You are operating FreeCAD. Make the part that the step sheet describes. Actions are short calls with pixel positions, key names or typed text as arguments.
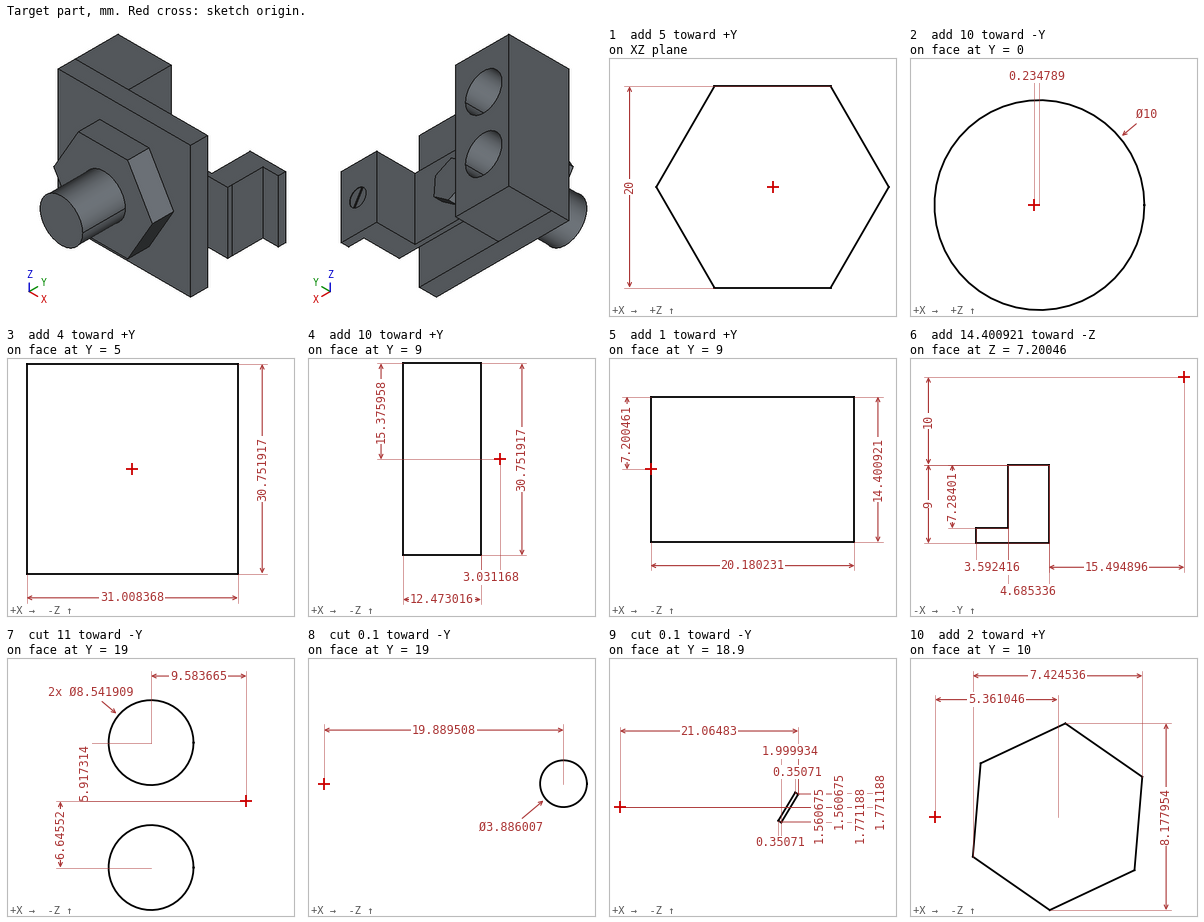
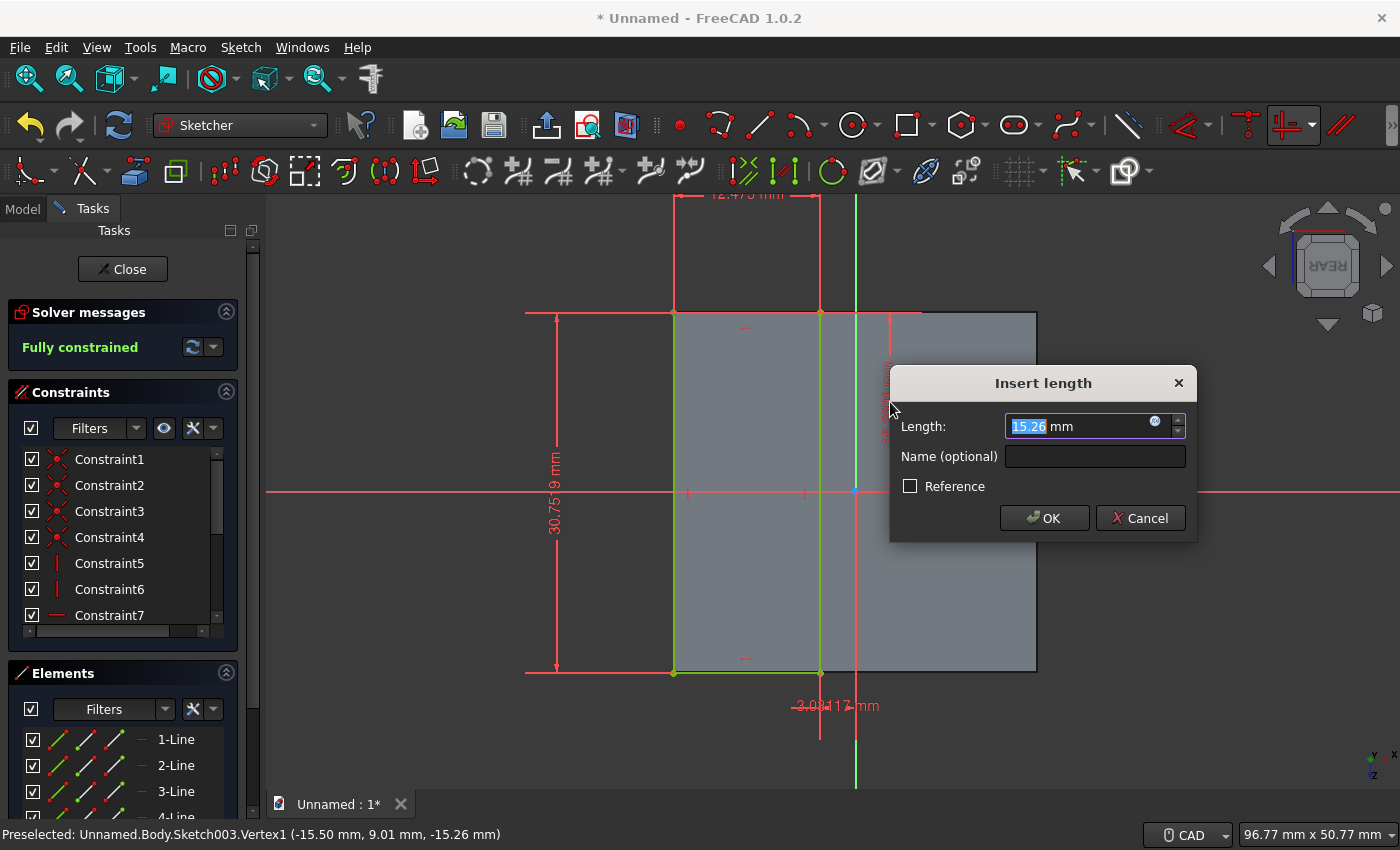
text(15.375958)
key(Return)
key(Escape)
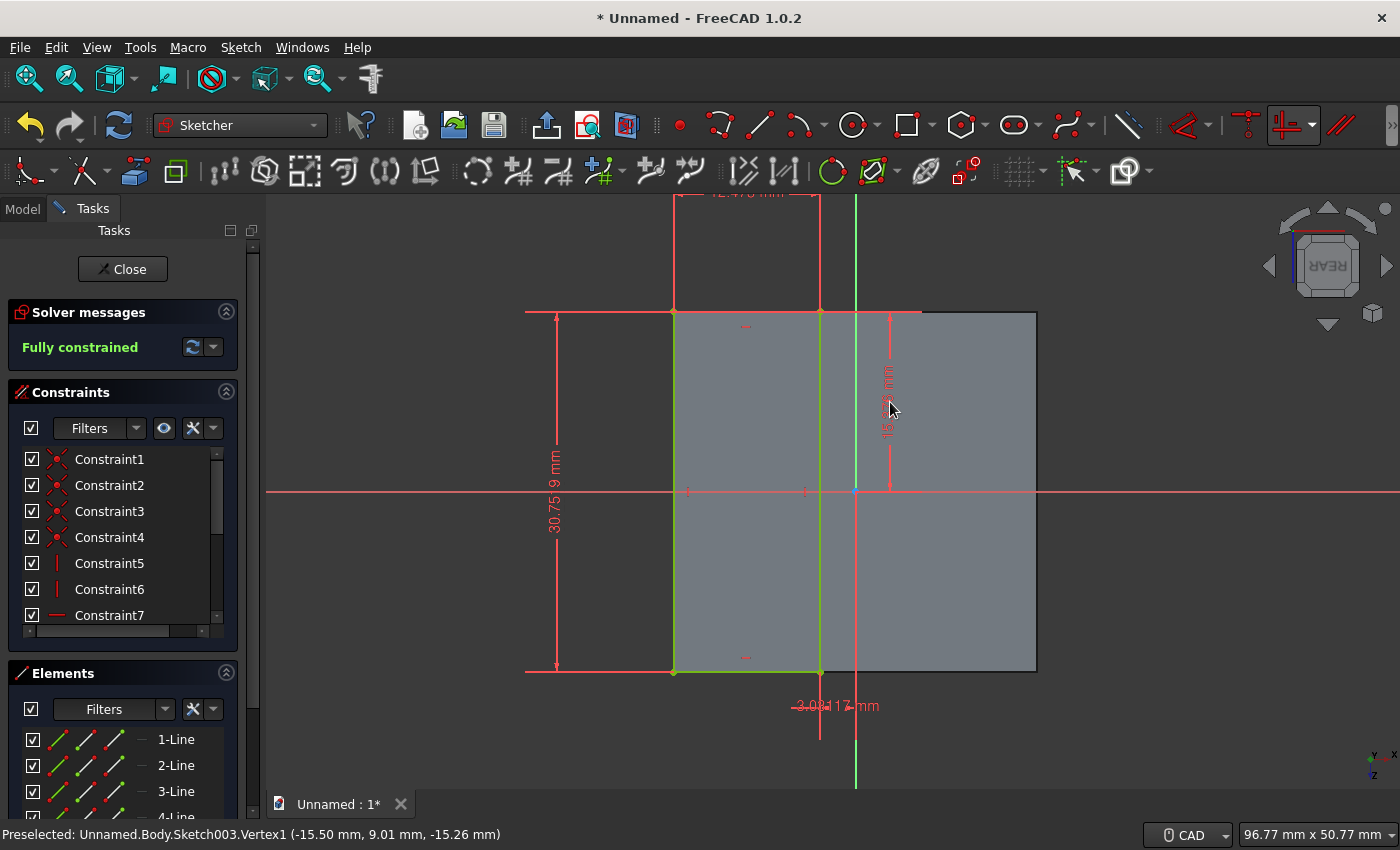
click(123, 269)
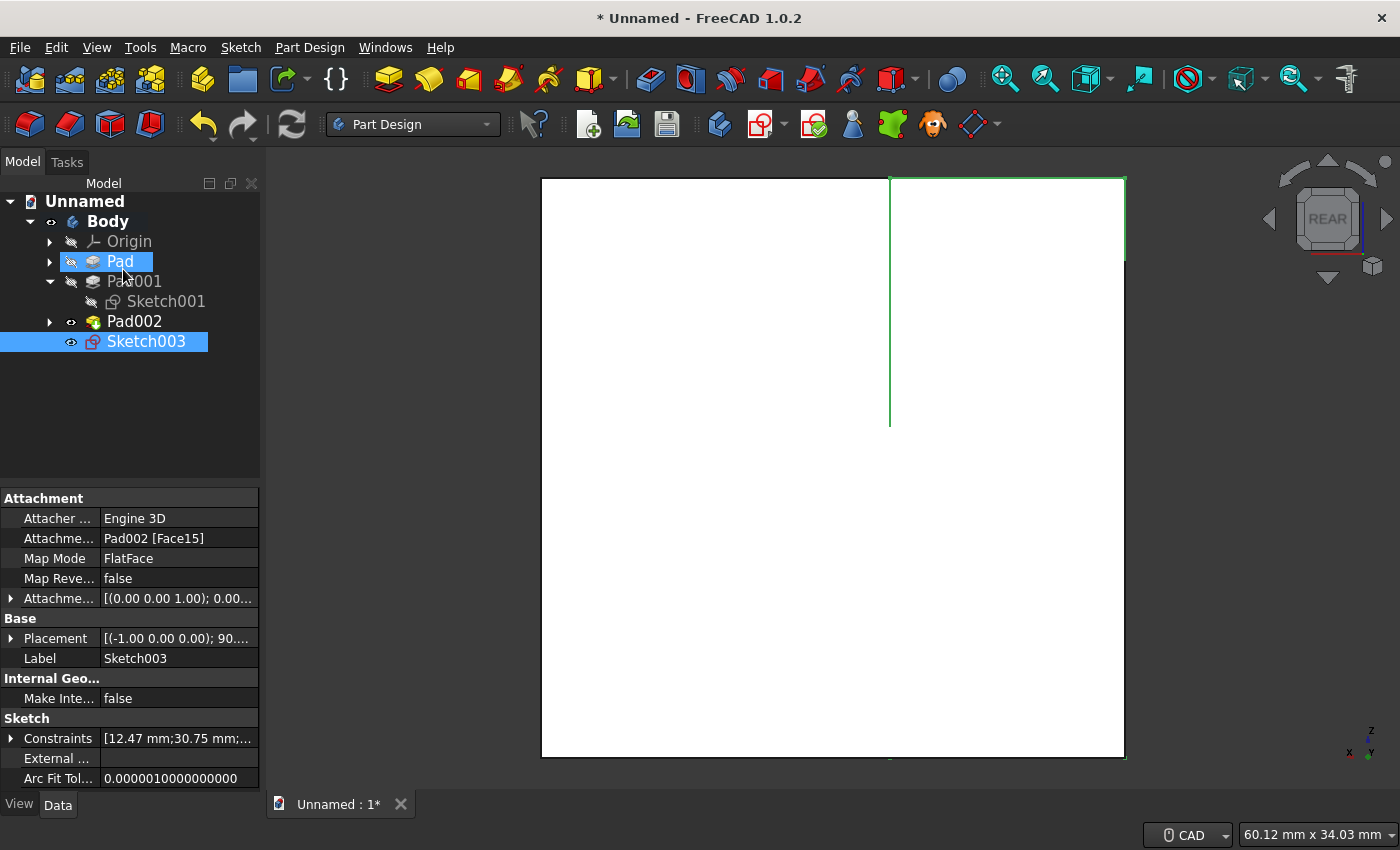
click(390, 80)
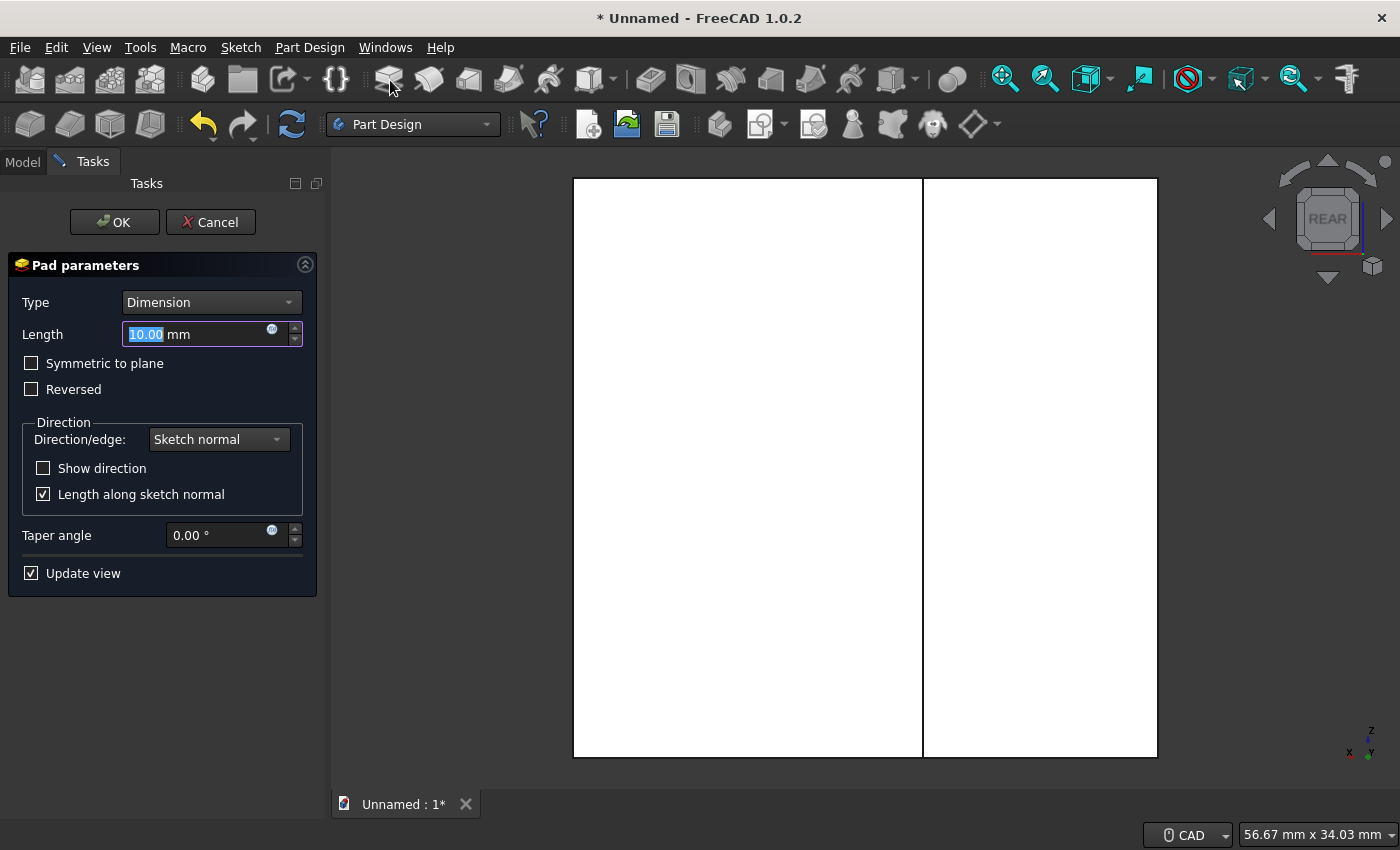
text(10)
key(Tab)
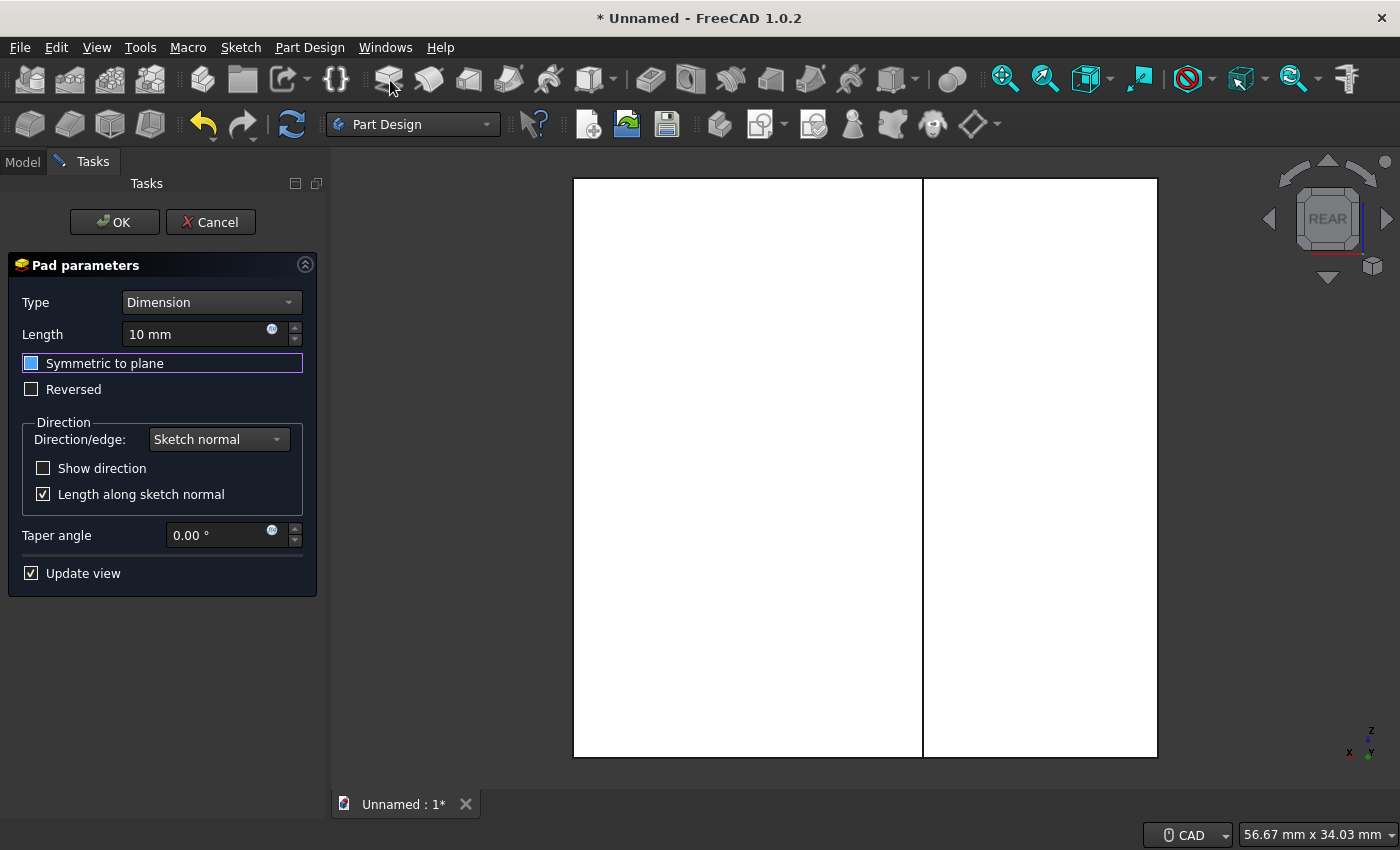
click(115, 222)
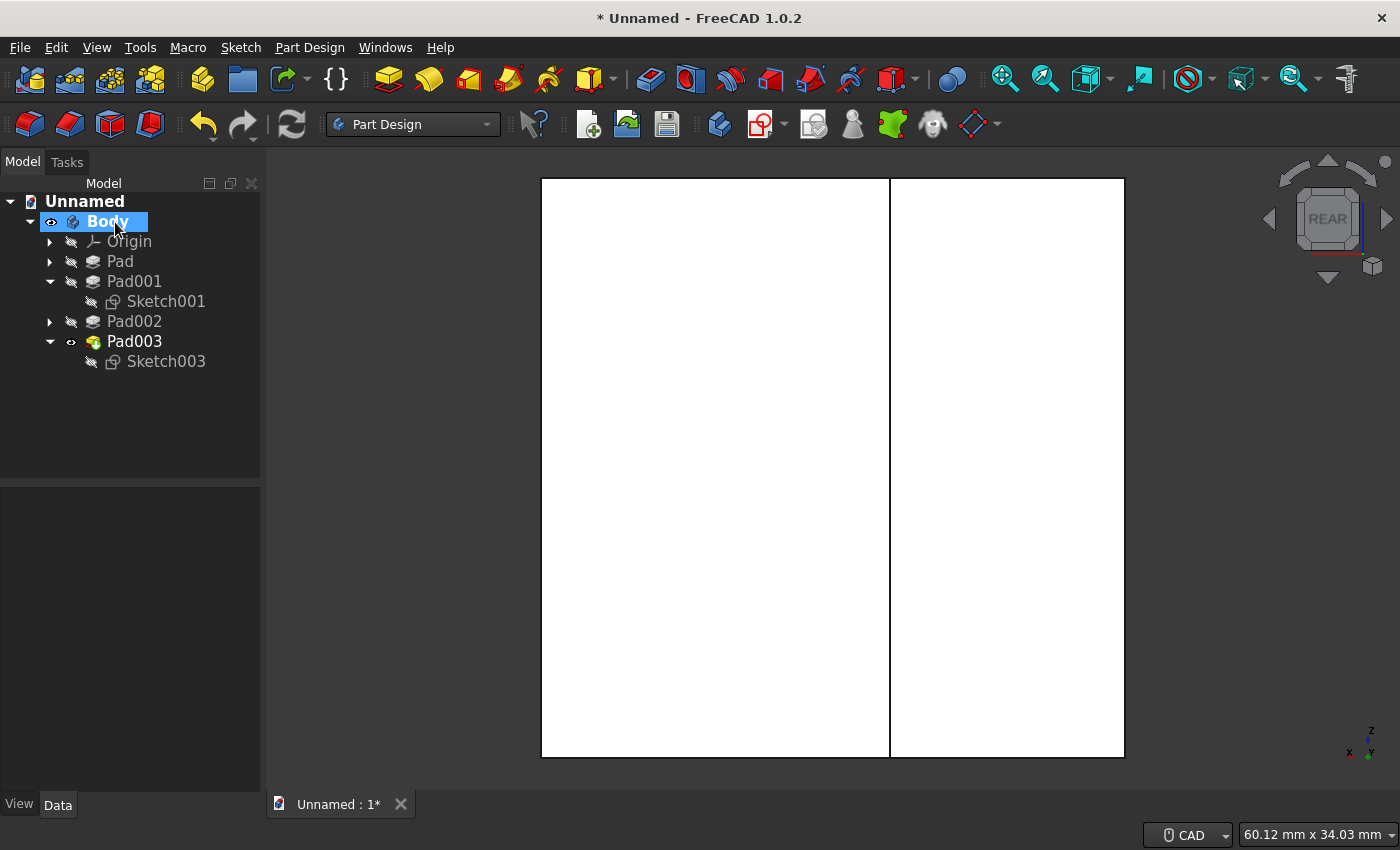
click(715, 550)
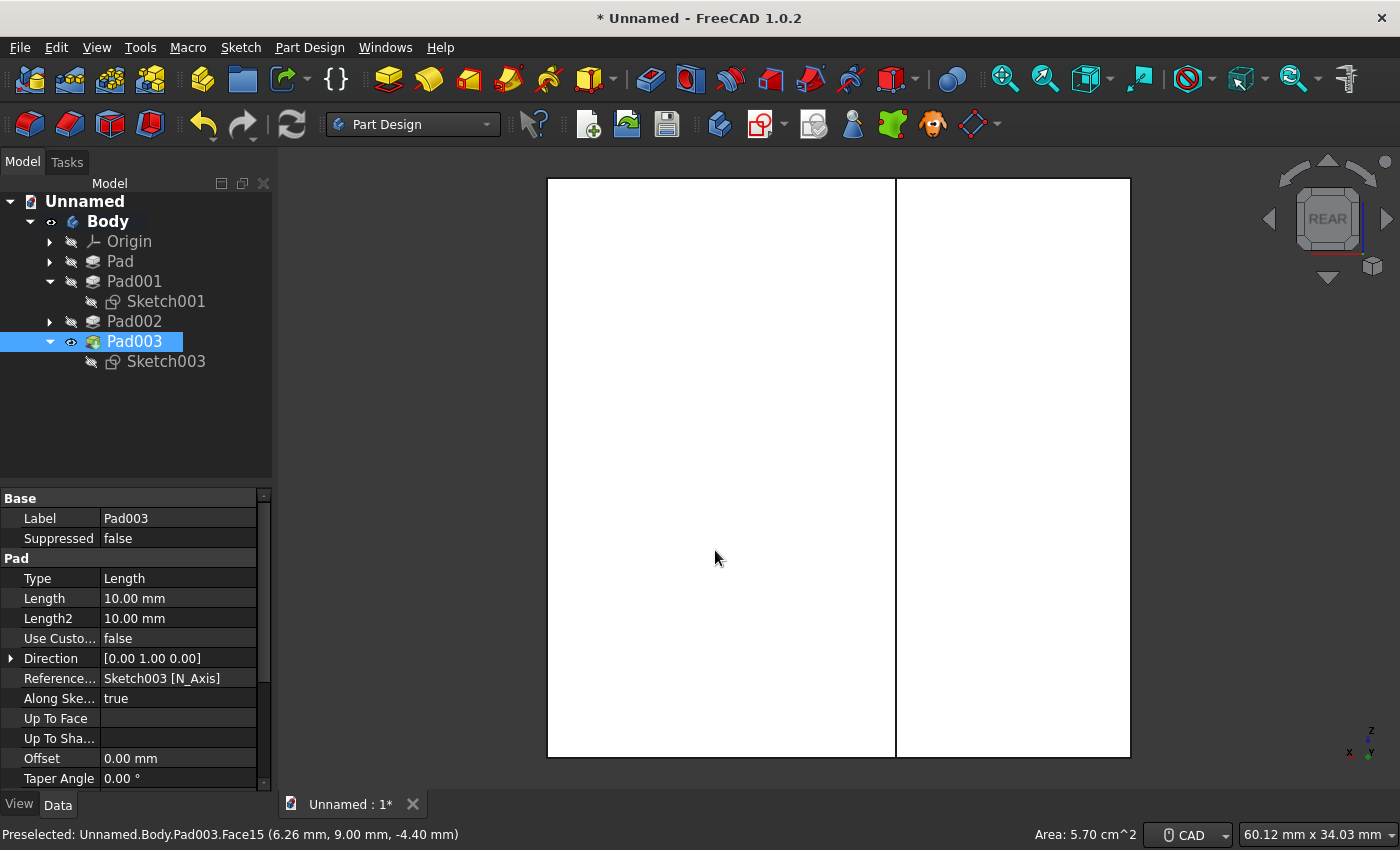
click(760, 124)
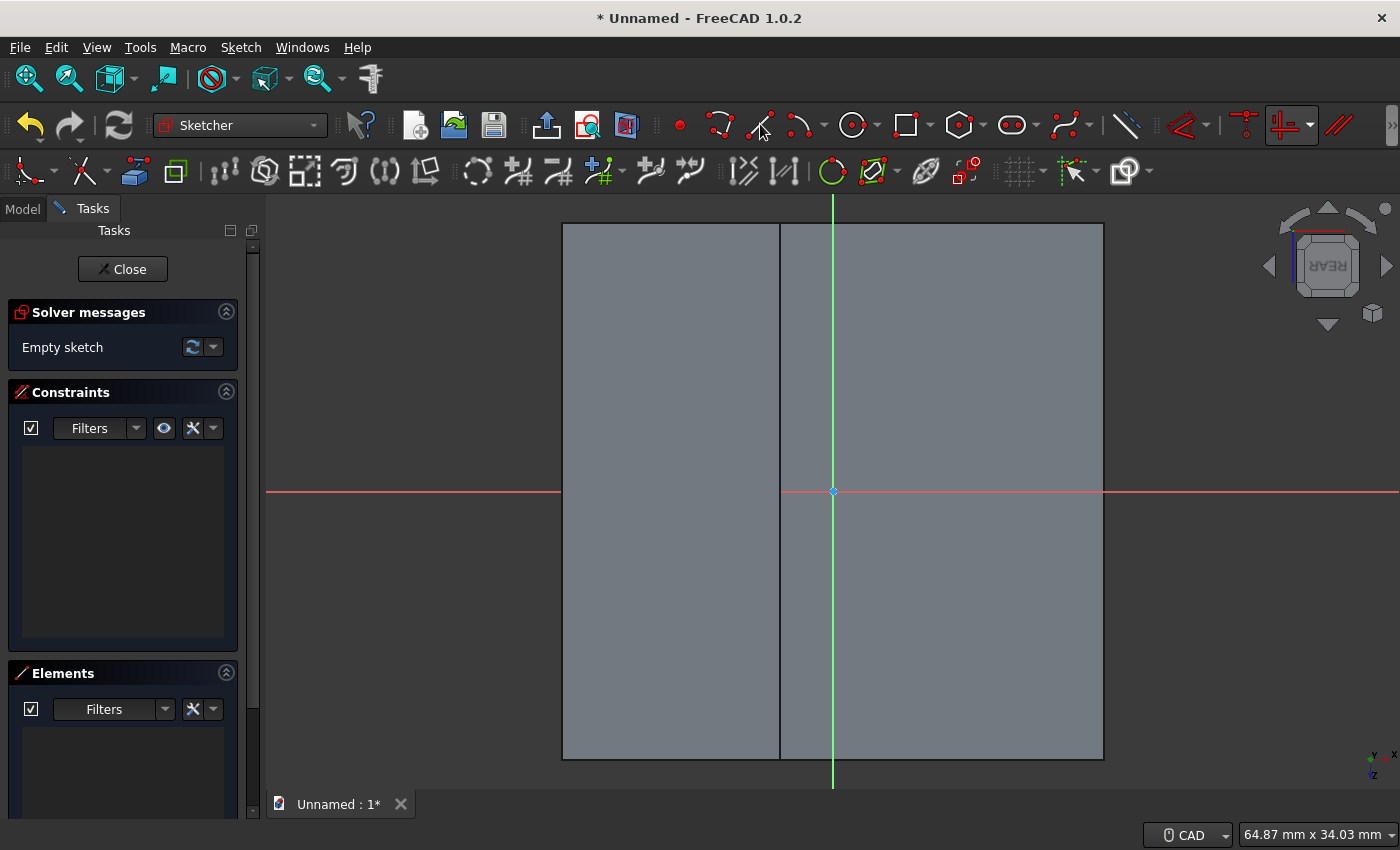
click(628, 126)